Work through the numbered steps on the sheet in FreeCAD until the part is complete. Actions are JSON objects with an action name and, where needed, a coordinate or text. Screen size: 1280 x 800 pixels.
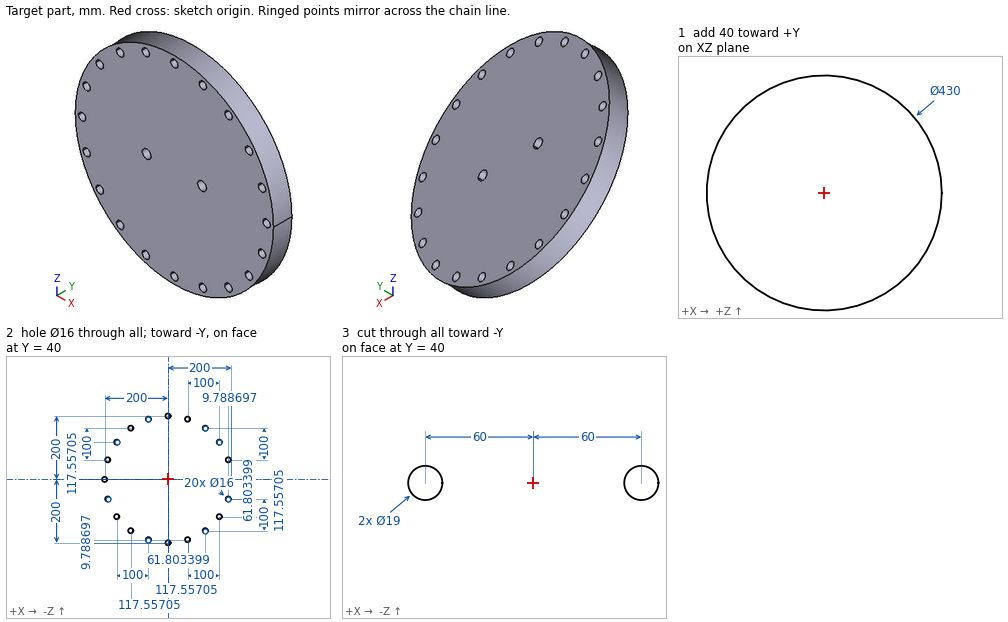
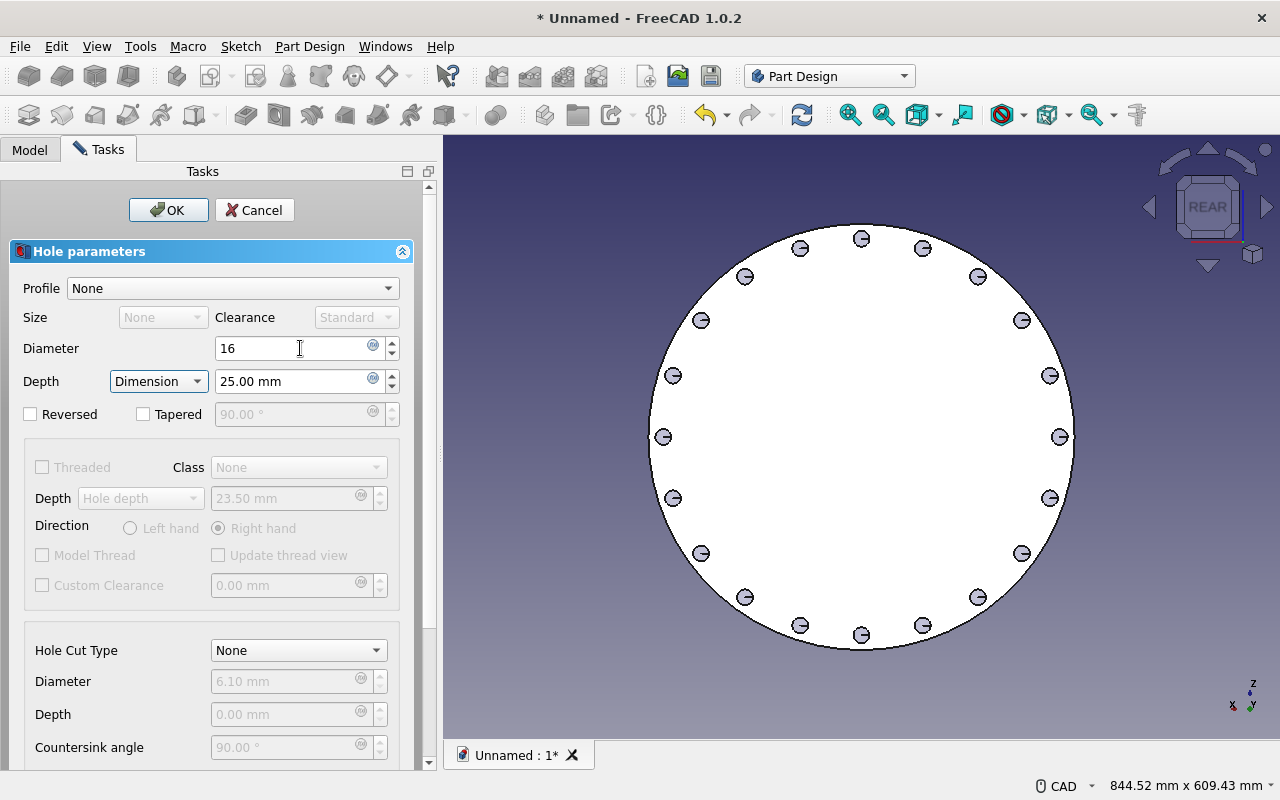
{"action": "left_click", "coordinate": [160, 382]}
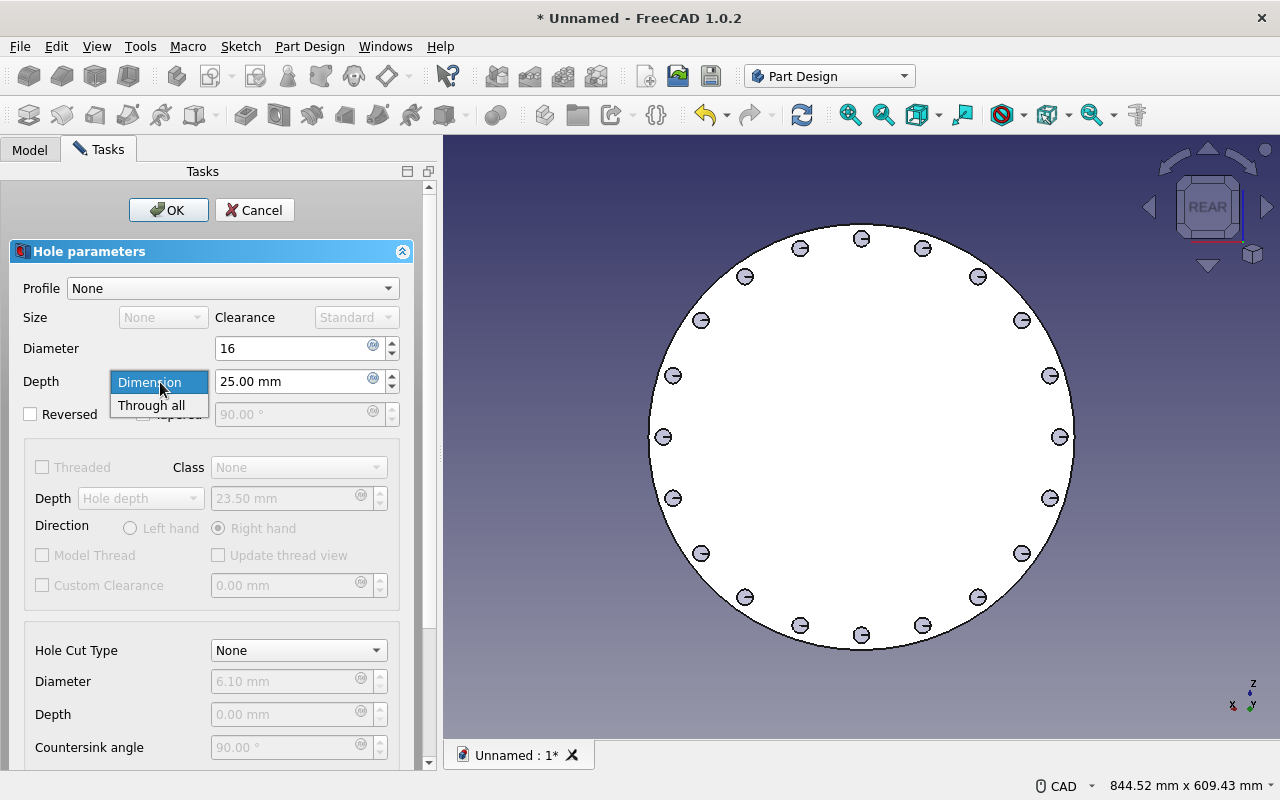
{"action": "left_click", "coordinate": [158, 406]}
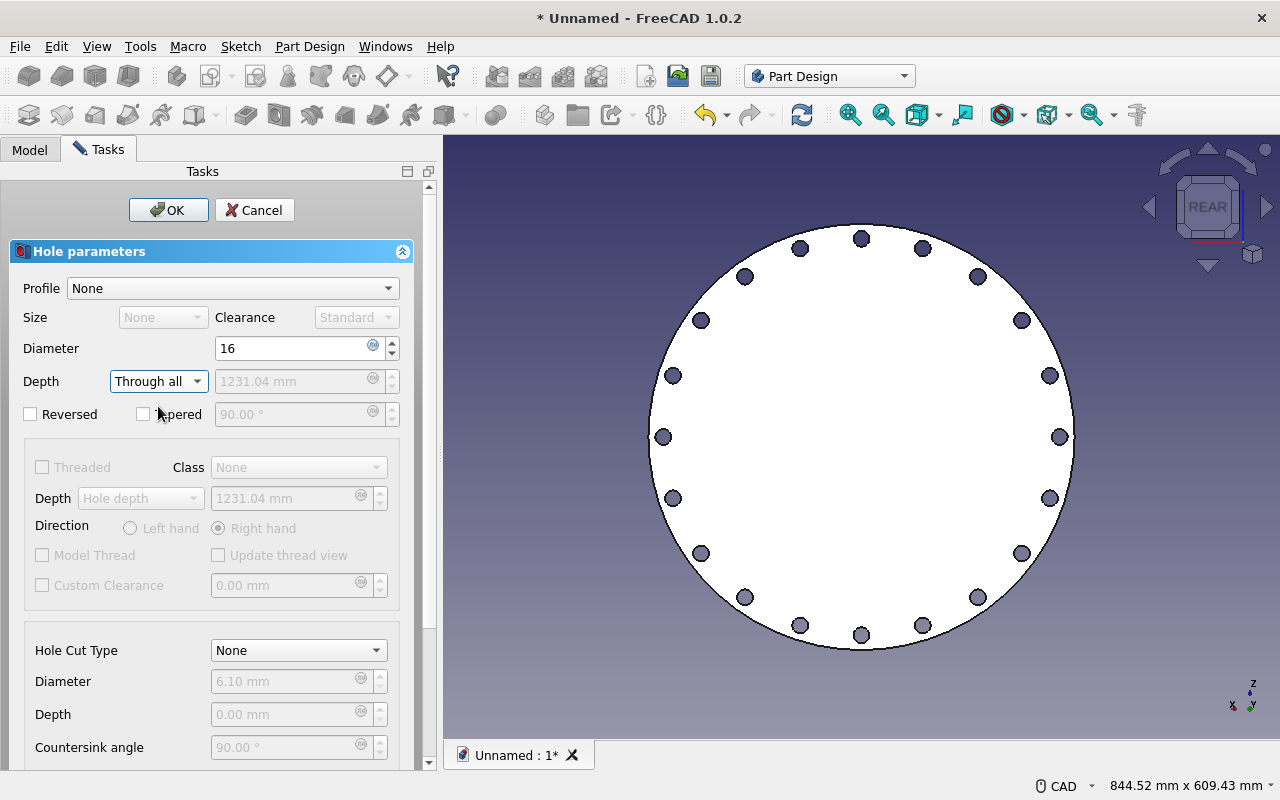
{"action": "left_click", "coordinate": [169, 210]}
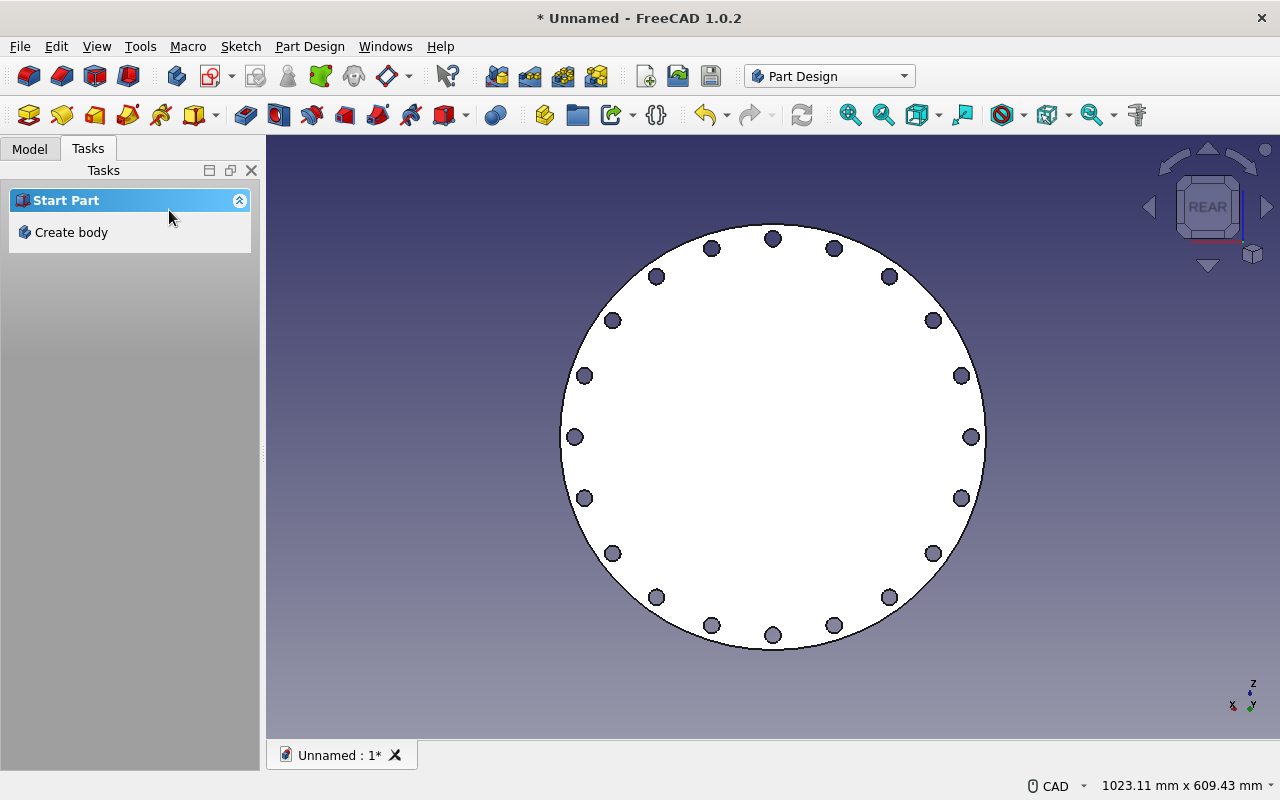
{"action": "left_click", "coordinate": [773, 436]}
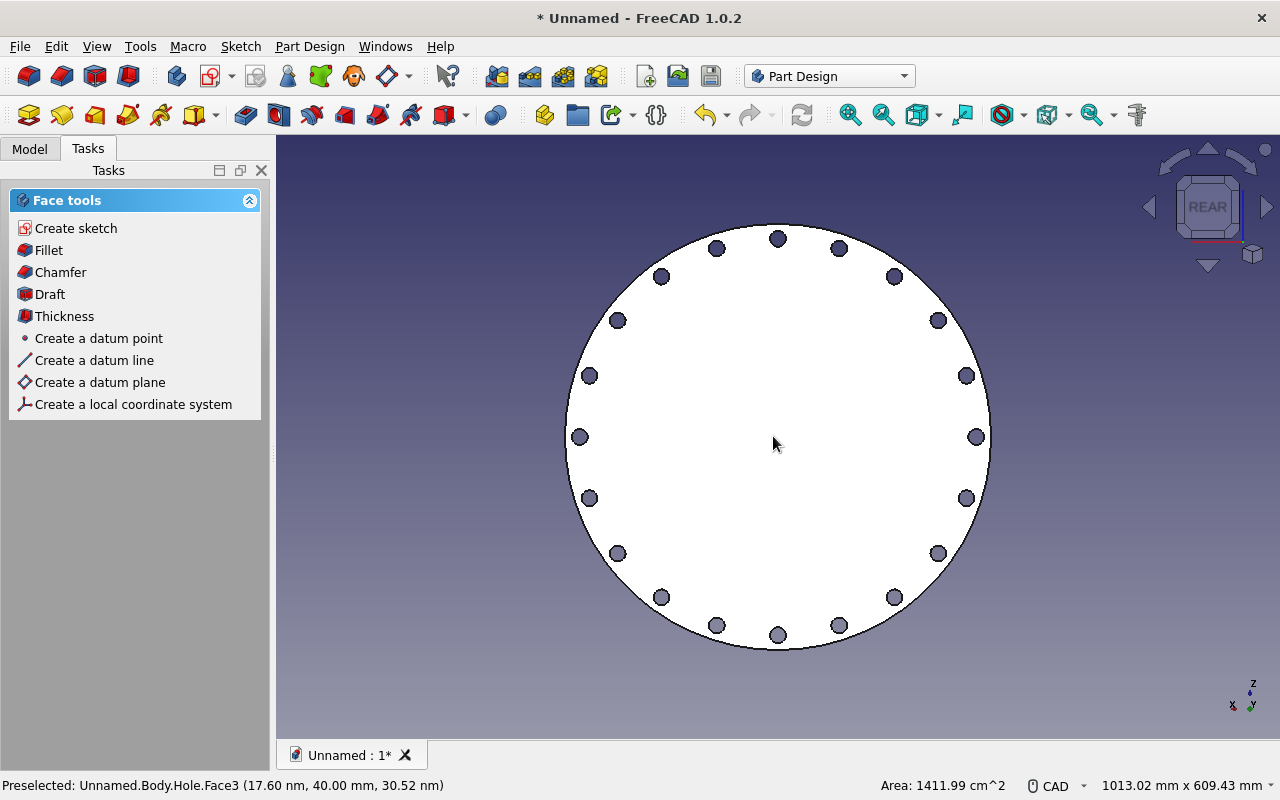
{"action": "left_click", "coordinate": [210, 76]}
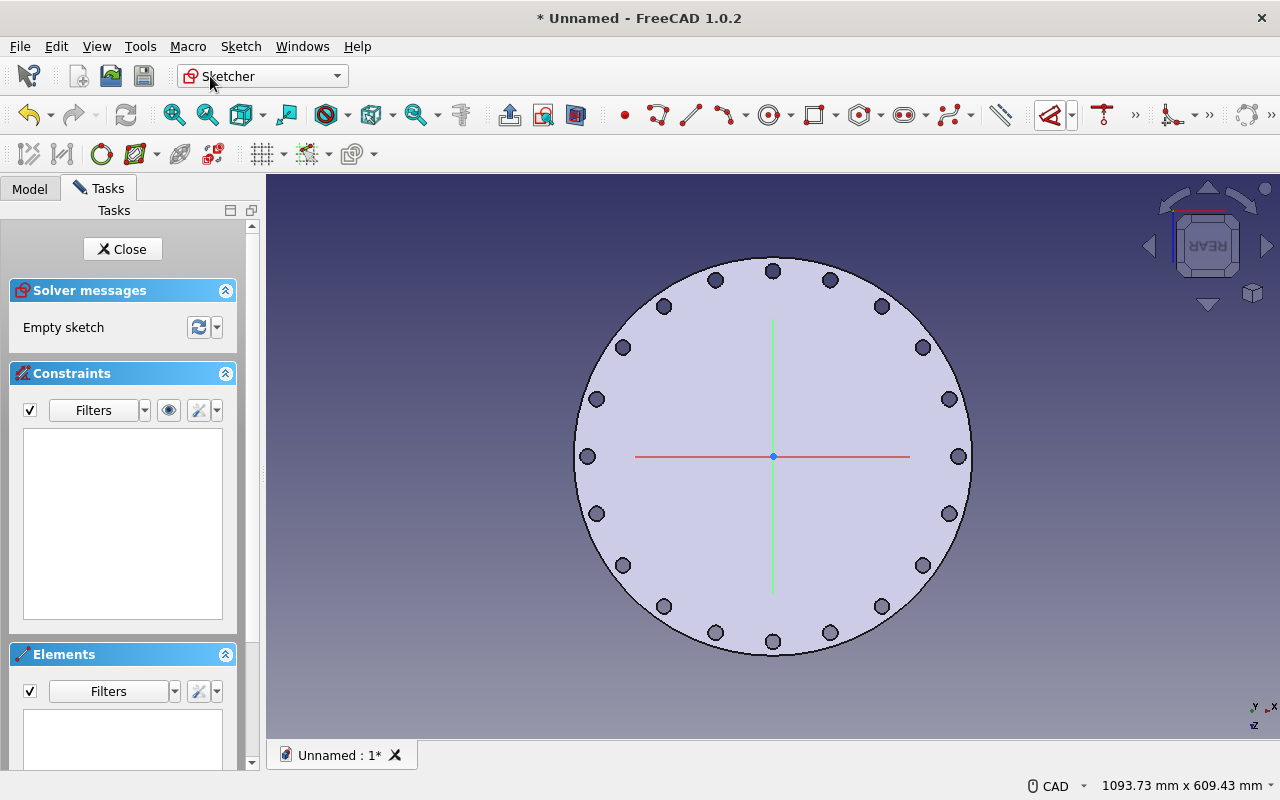
{"action": "scroll", "coordinate": [790, 456], "scroll_direction": "up", "scroll_amount": 8}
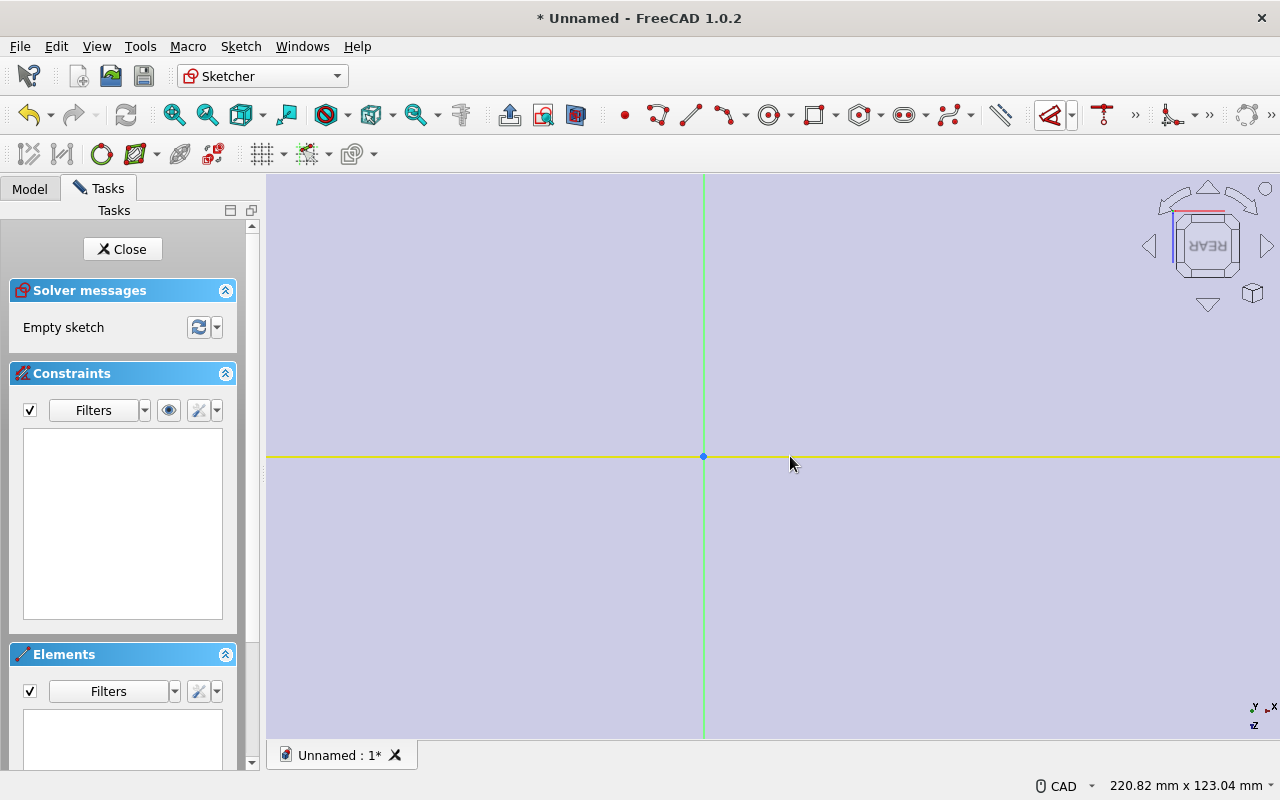
{"action": "key", "text": "g c"}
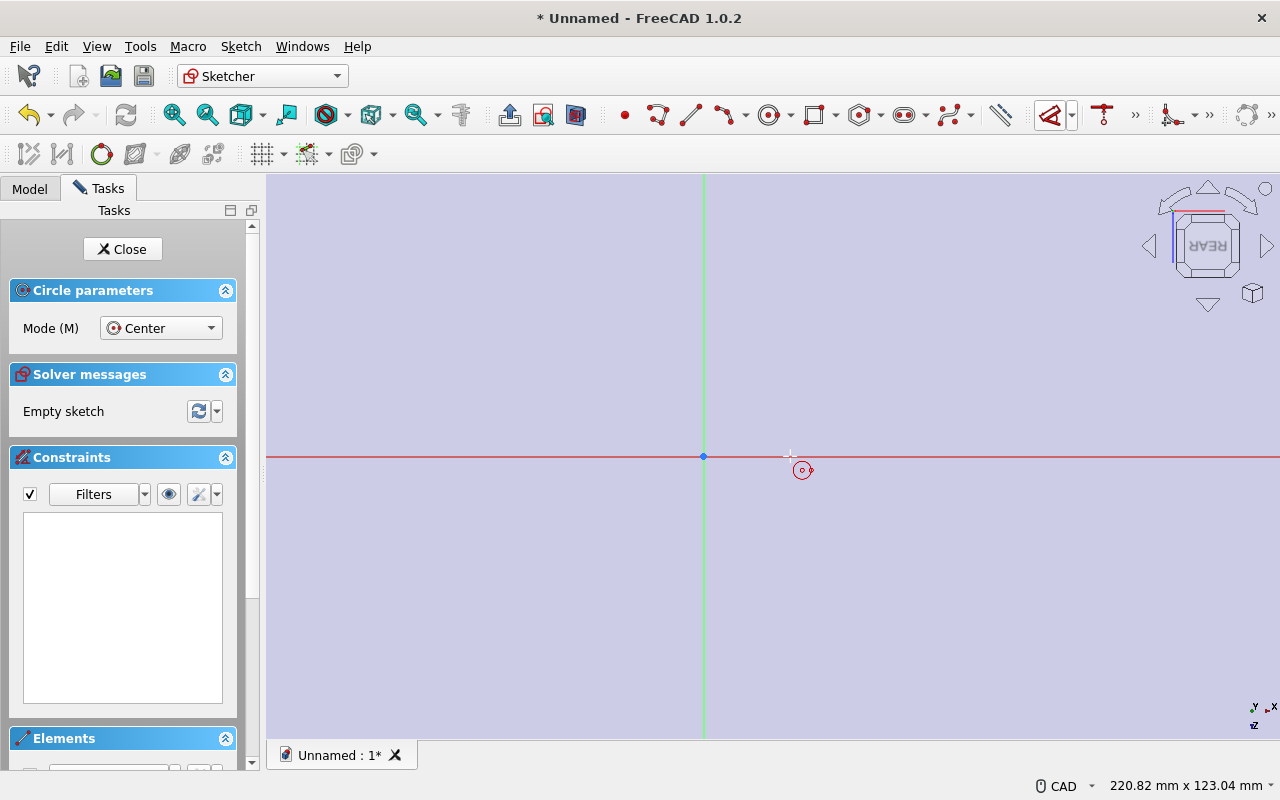
{"action": "left_click", "coordinate": [428, 456]}
{"action": "left_click", "coordinate": [459, 426]}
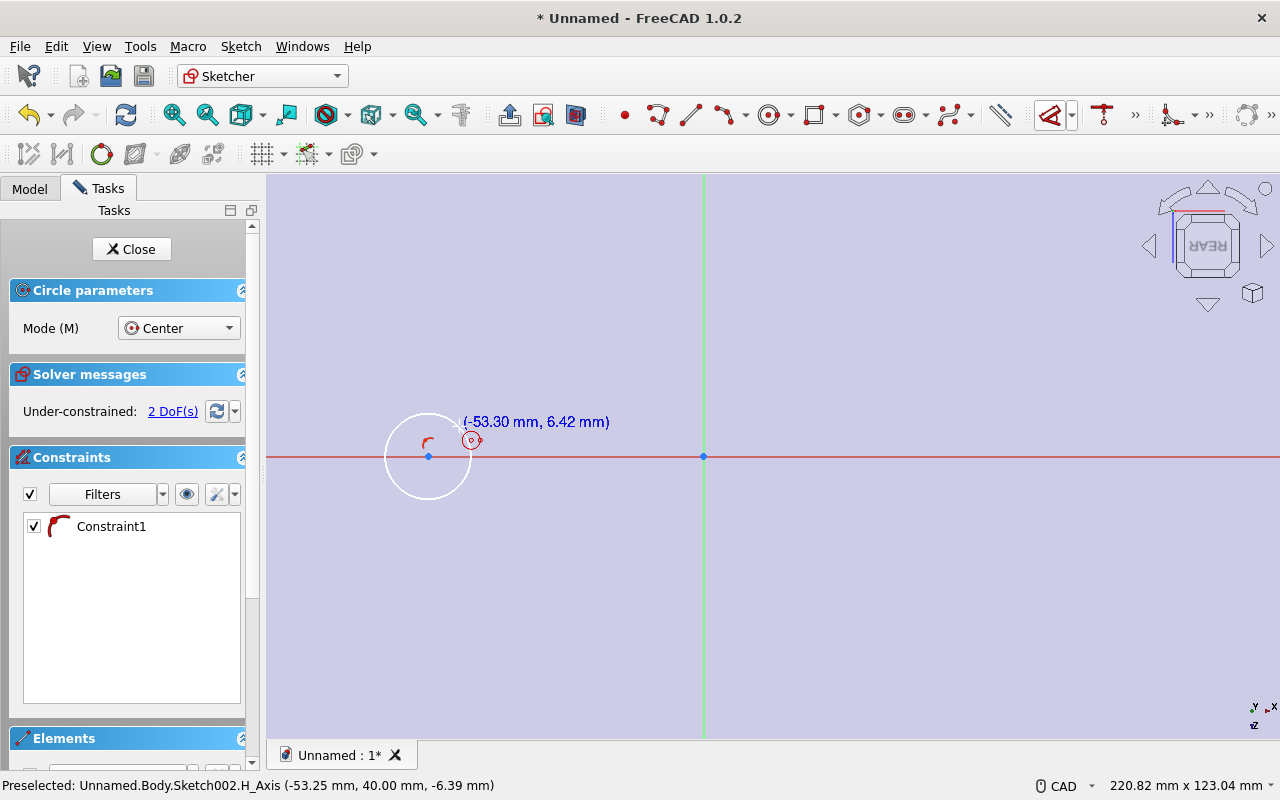
{"action": "left_click", "coordinate": [979, 456]}
{"action": "left_click", "coordinate": [1010, 426]}
{"action": "key", "text": "Escape"}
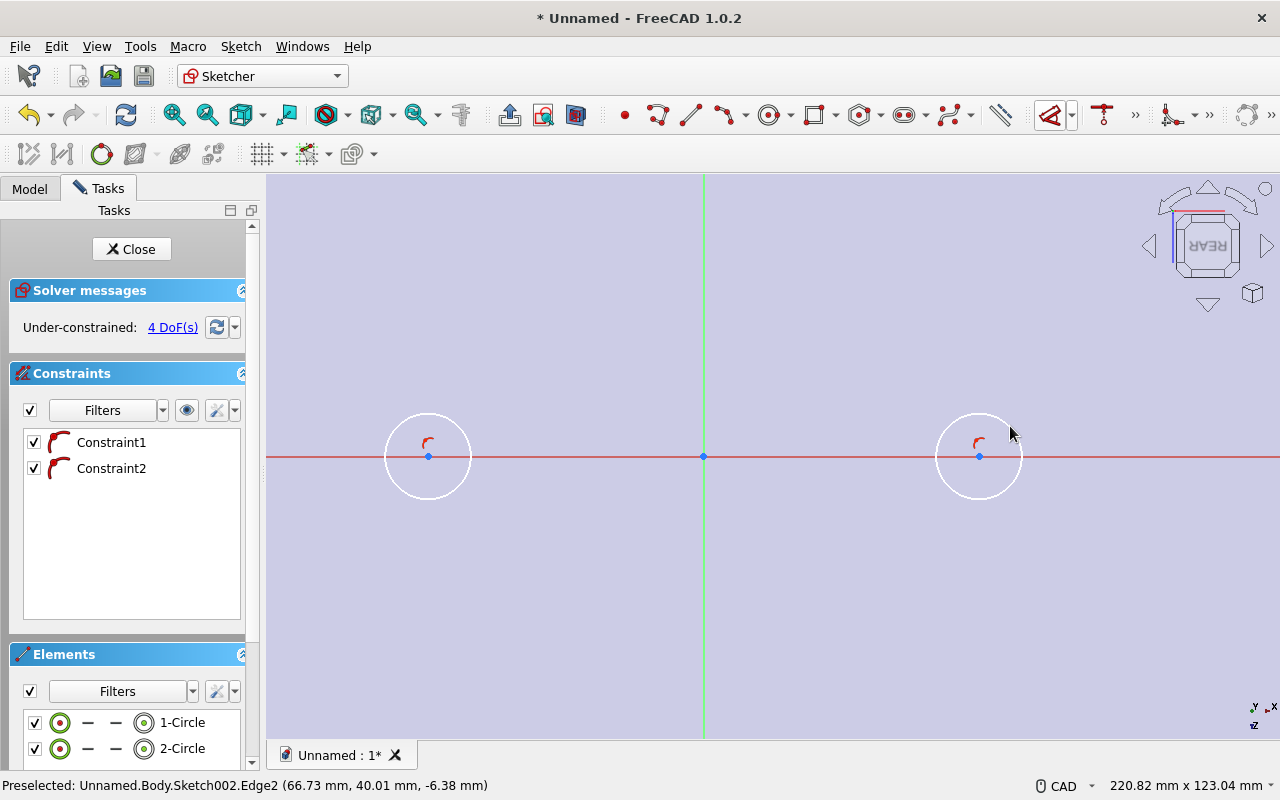
{"action": "left_click", "coordinate": [458, 426]}